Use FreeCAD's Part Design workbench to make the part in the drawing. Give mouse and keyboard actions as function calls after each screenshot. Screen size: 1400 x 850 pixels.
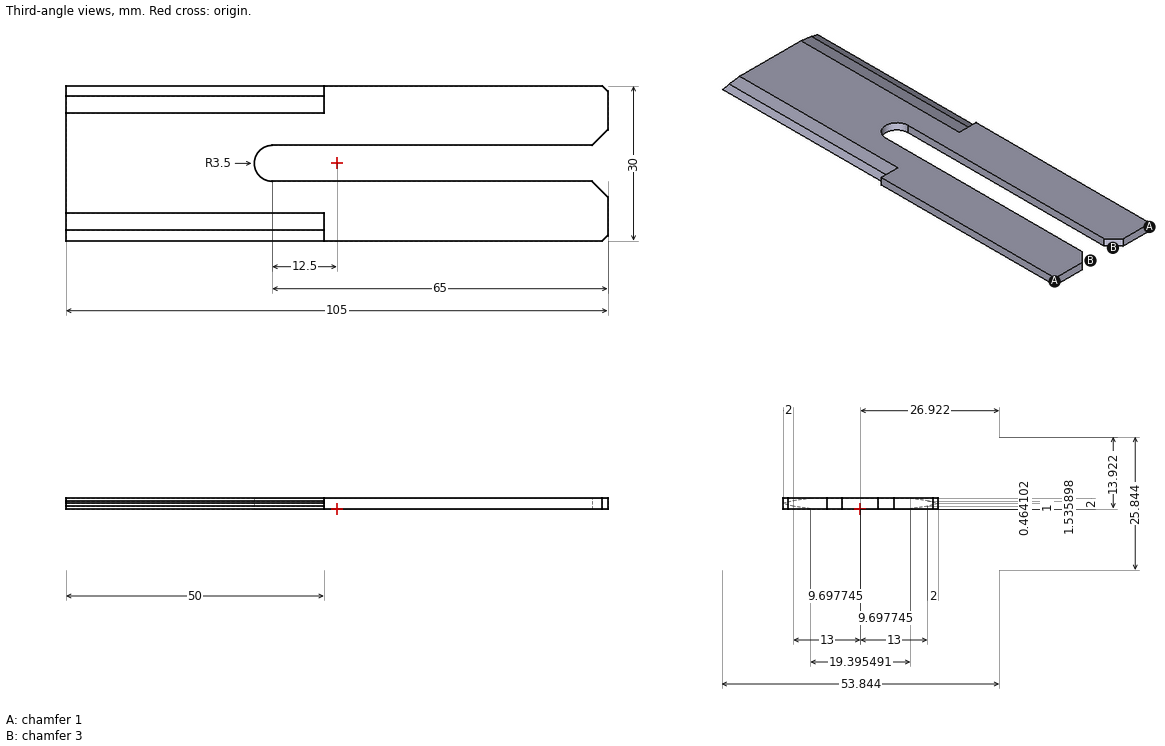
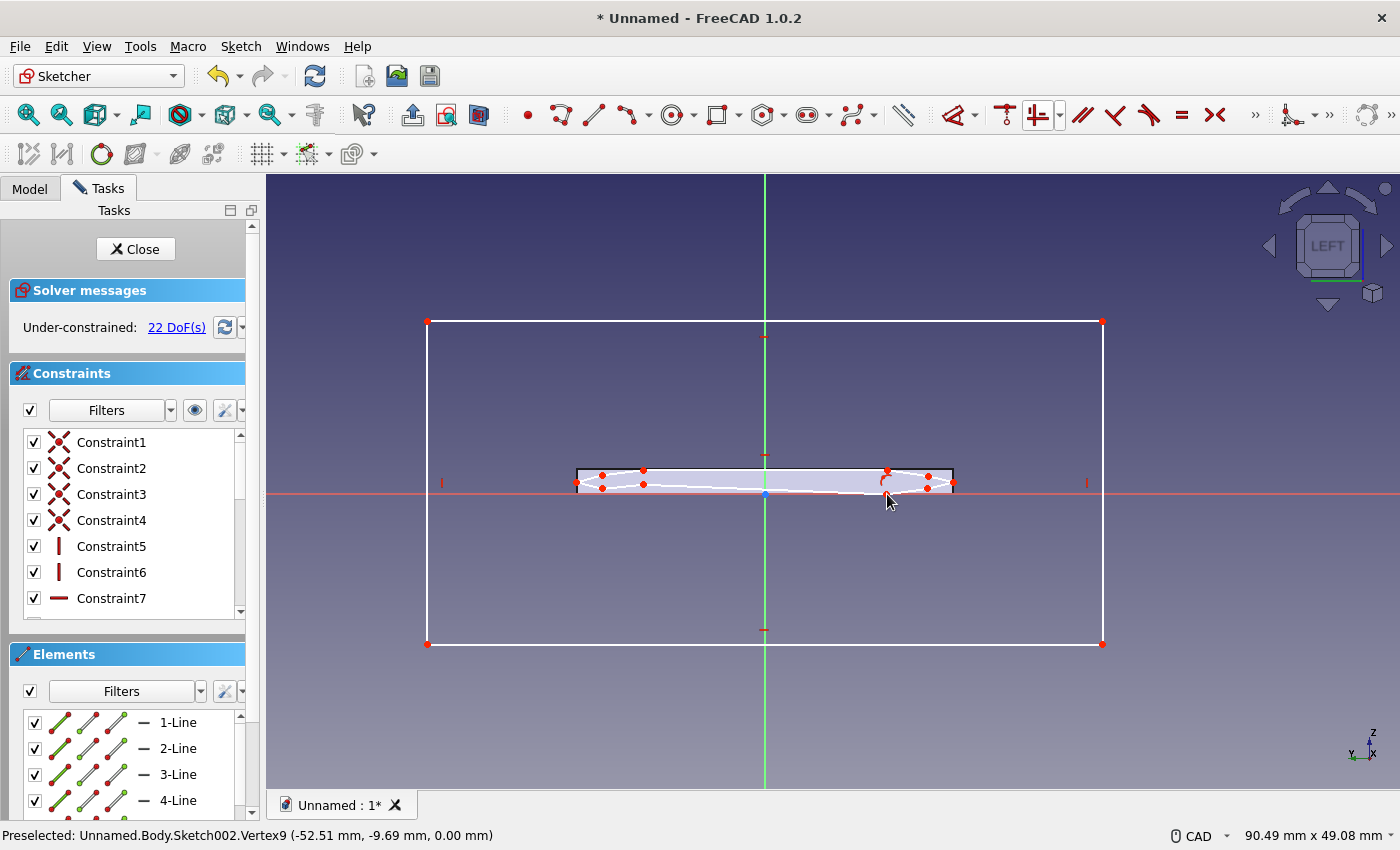
click(814, 492)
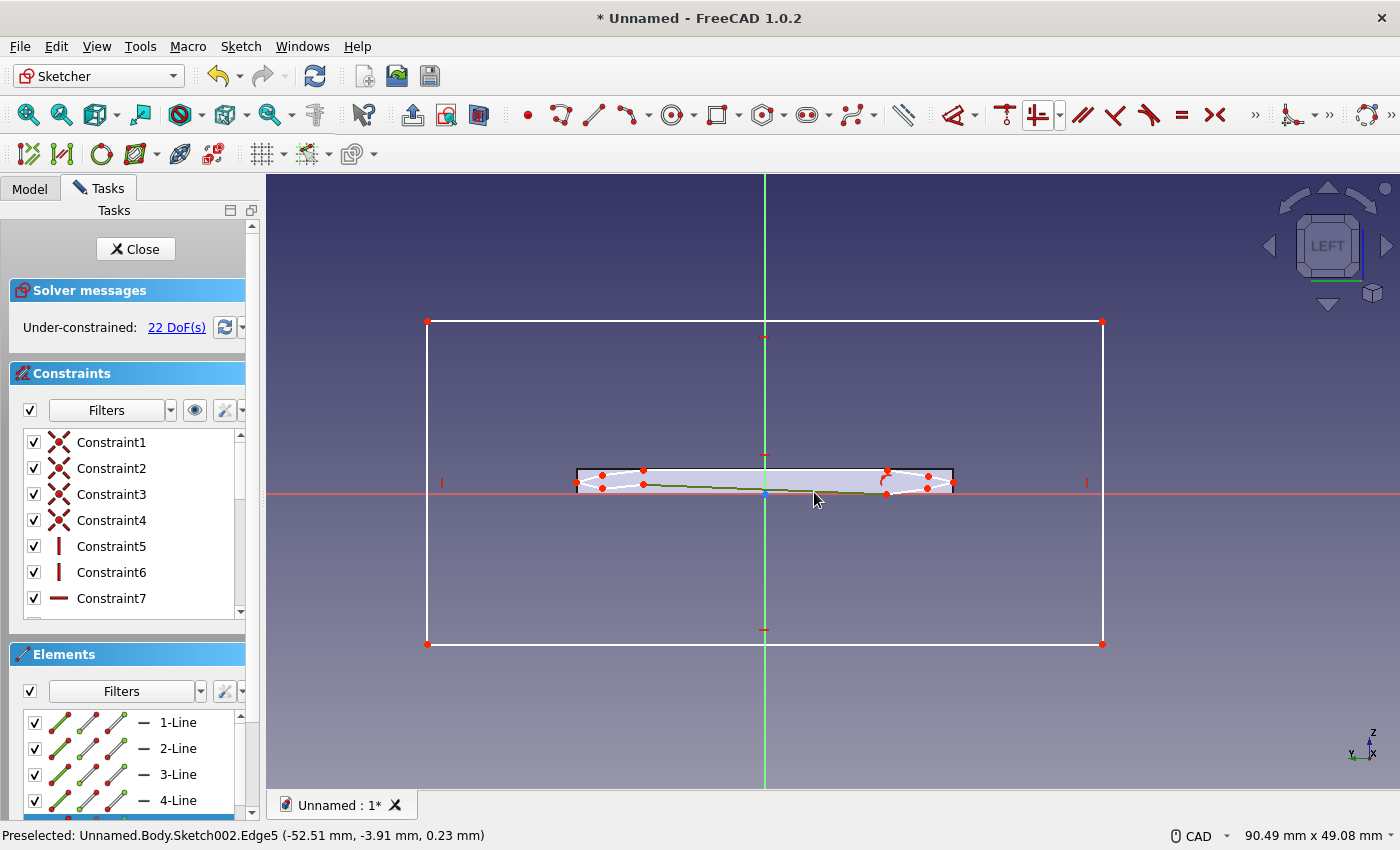
click(1060, 116)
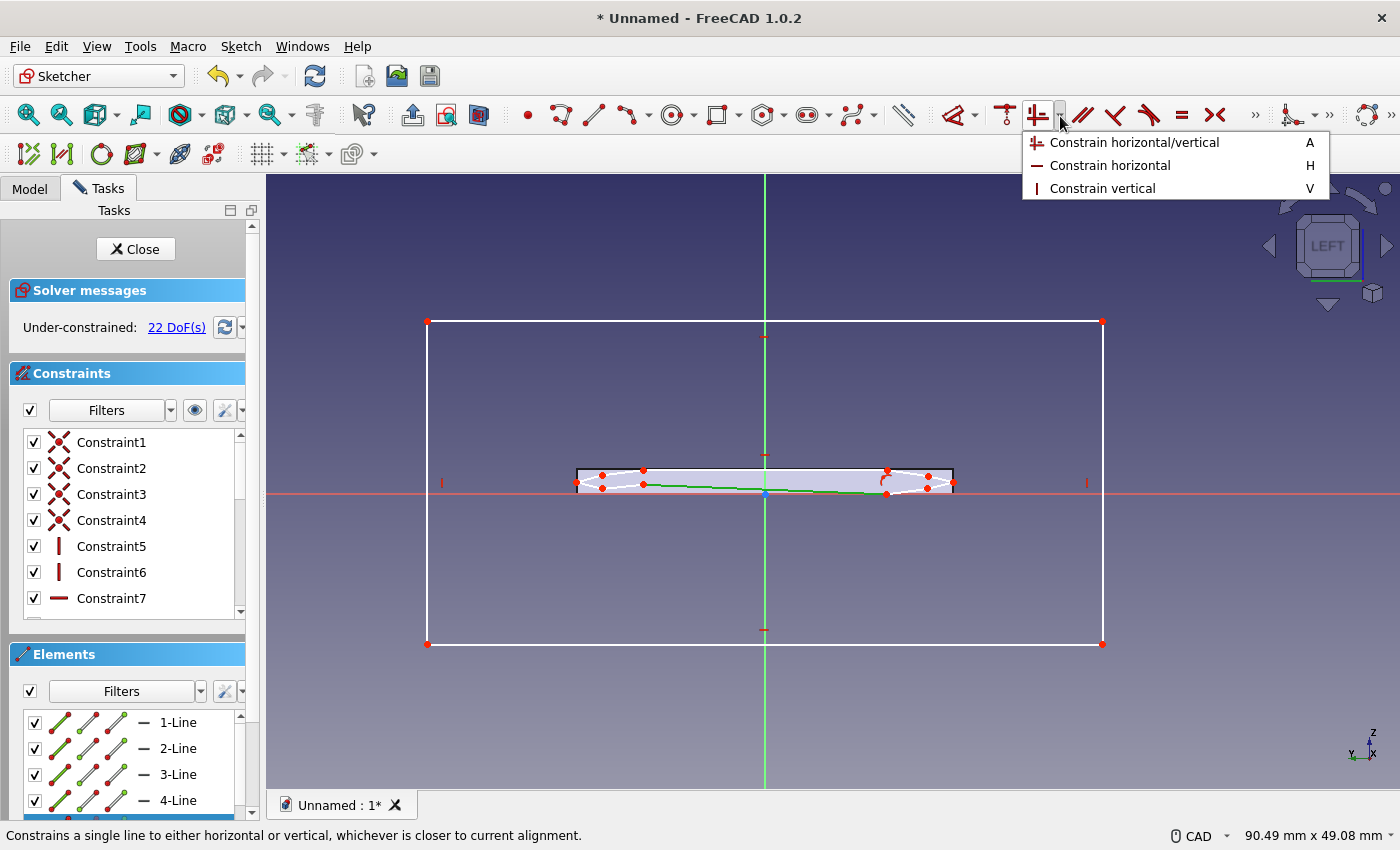
click(1176, 166)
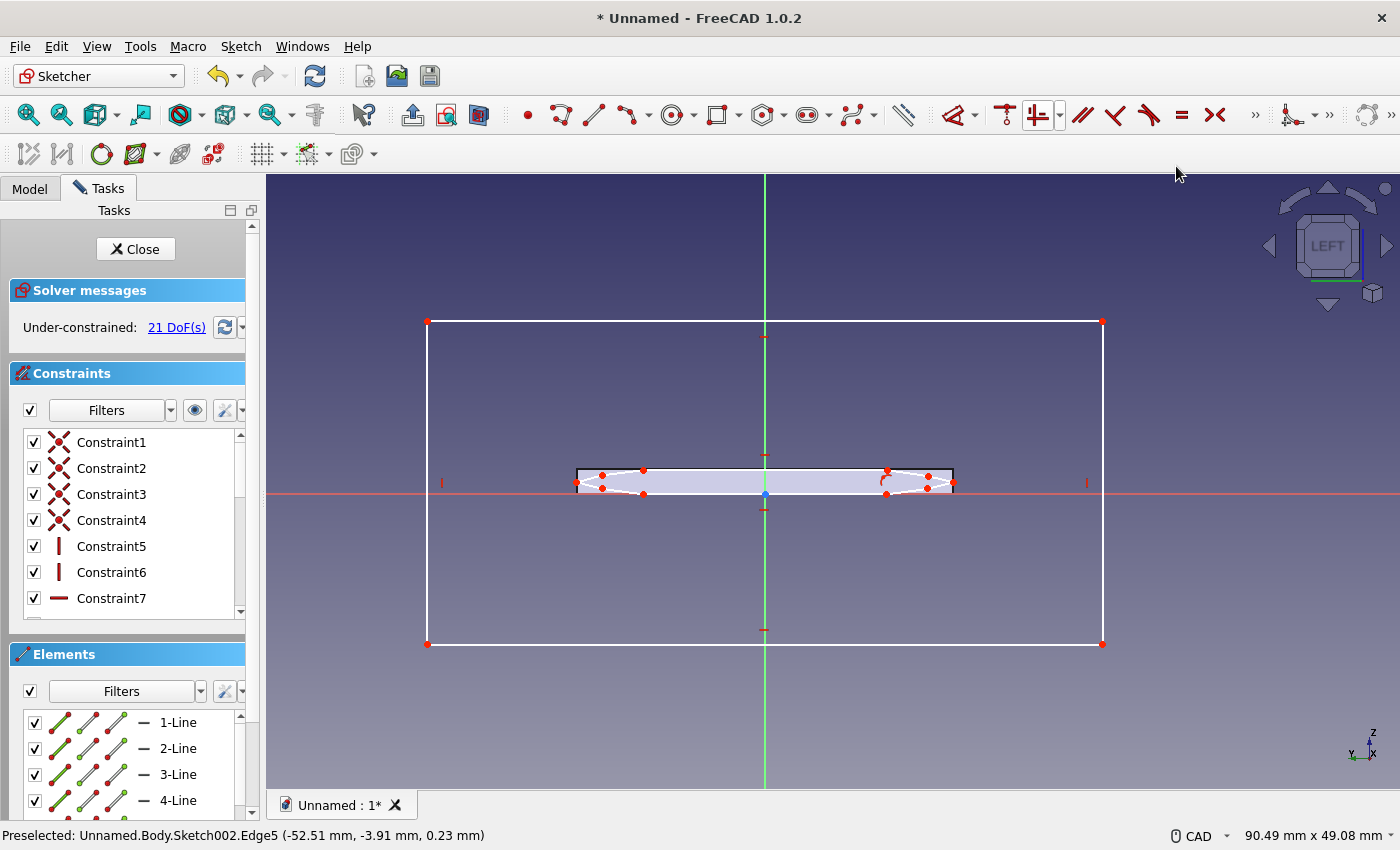
click(952, 116)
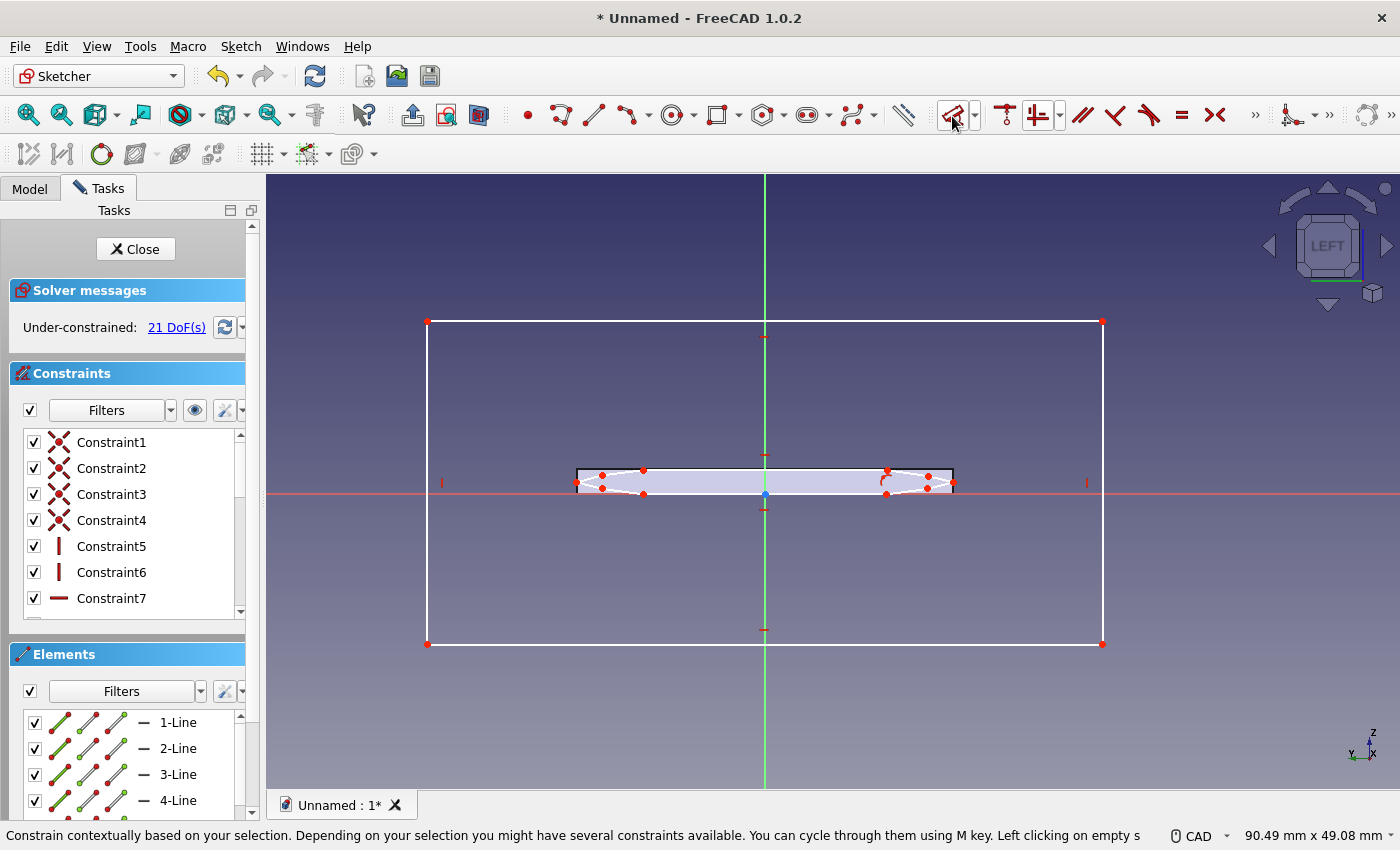
scroll(577, 482, up, 6)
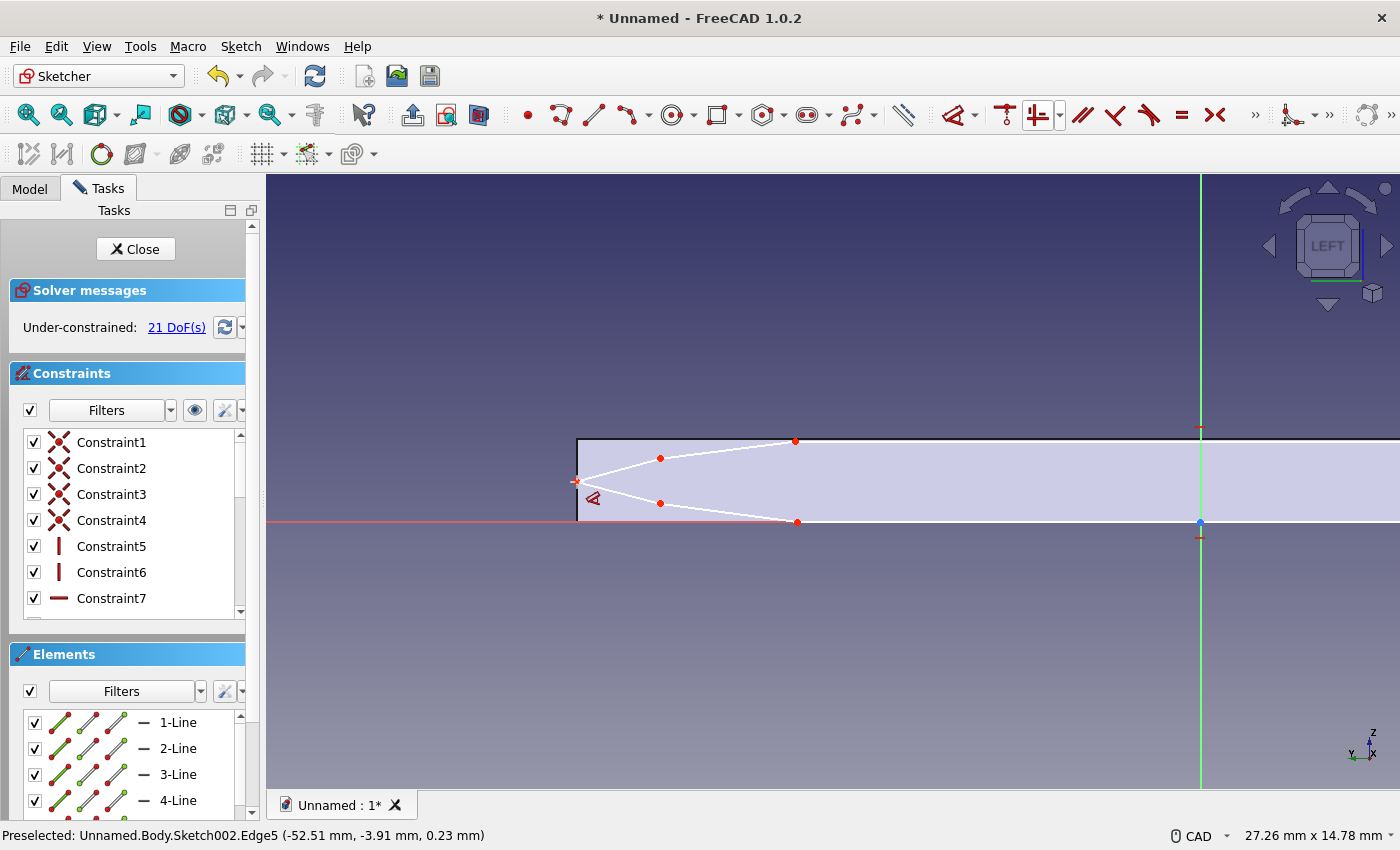
click(576, 482)
click(542, 502)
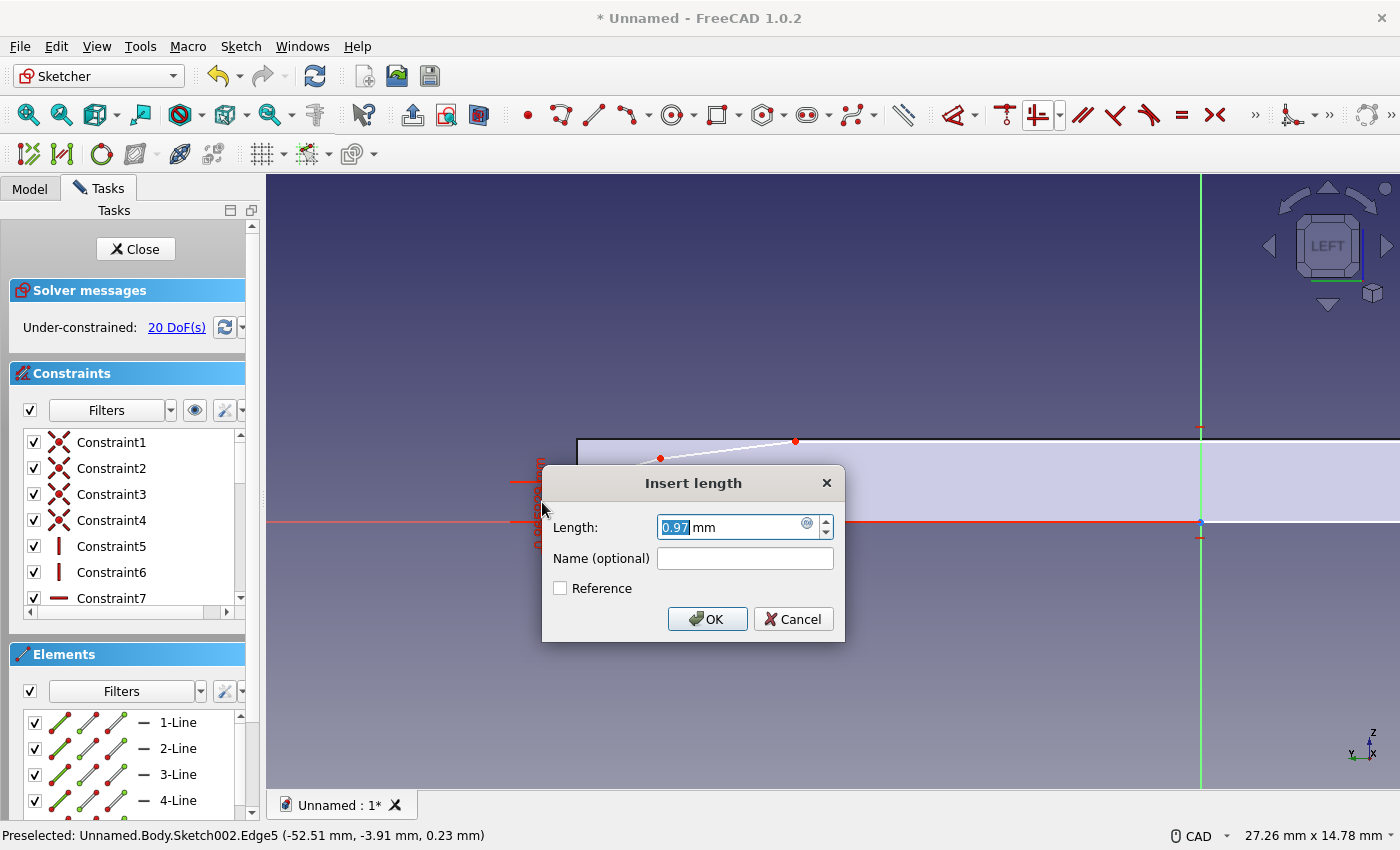
text(1)
key(Return)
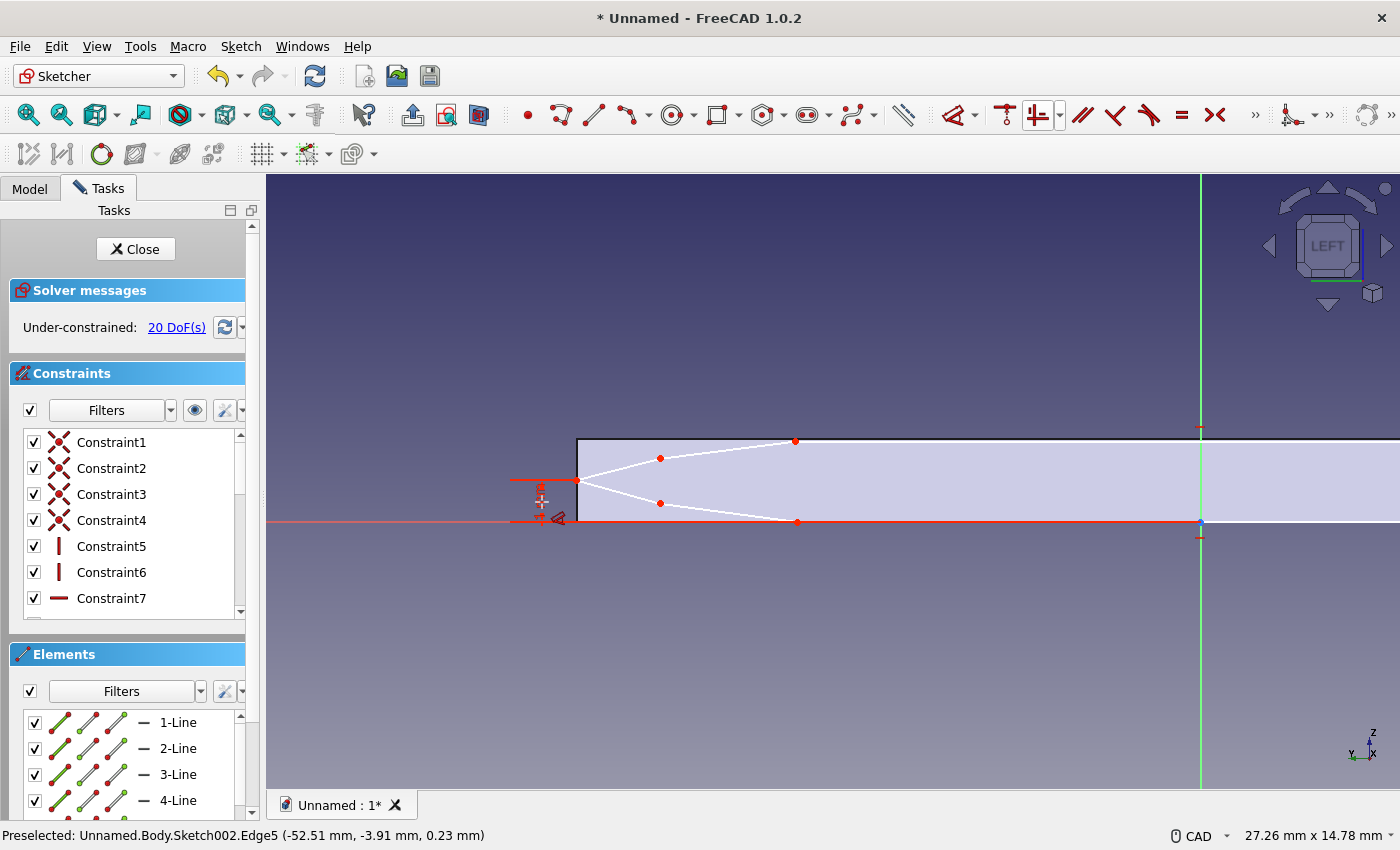
click(796, 442)
click(762, 482)